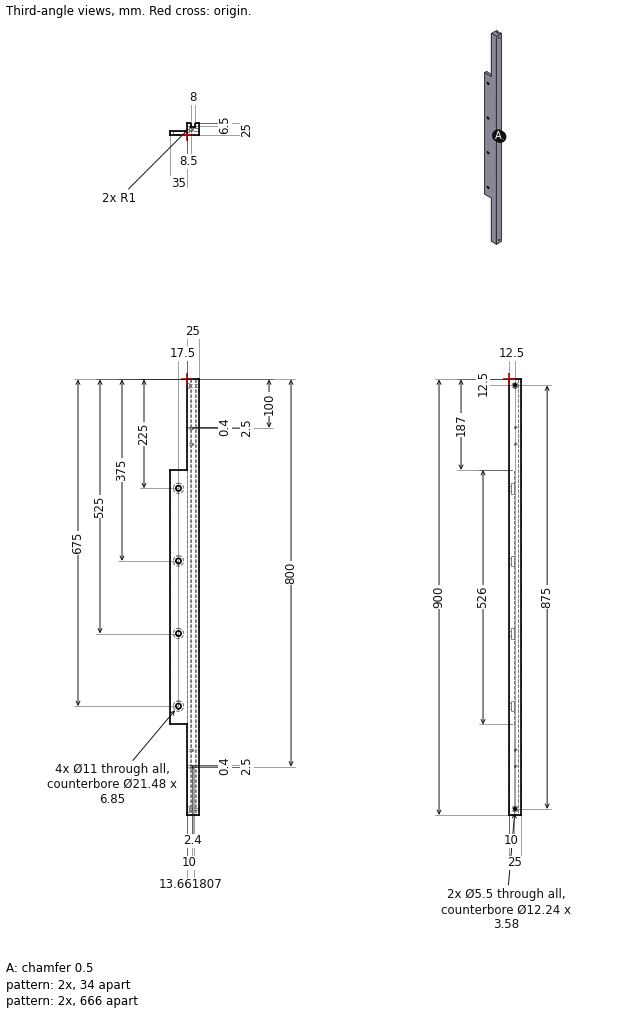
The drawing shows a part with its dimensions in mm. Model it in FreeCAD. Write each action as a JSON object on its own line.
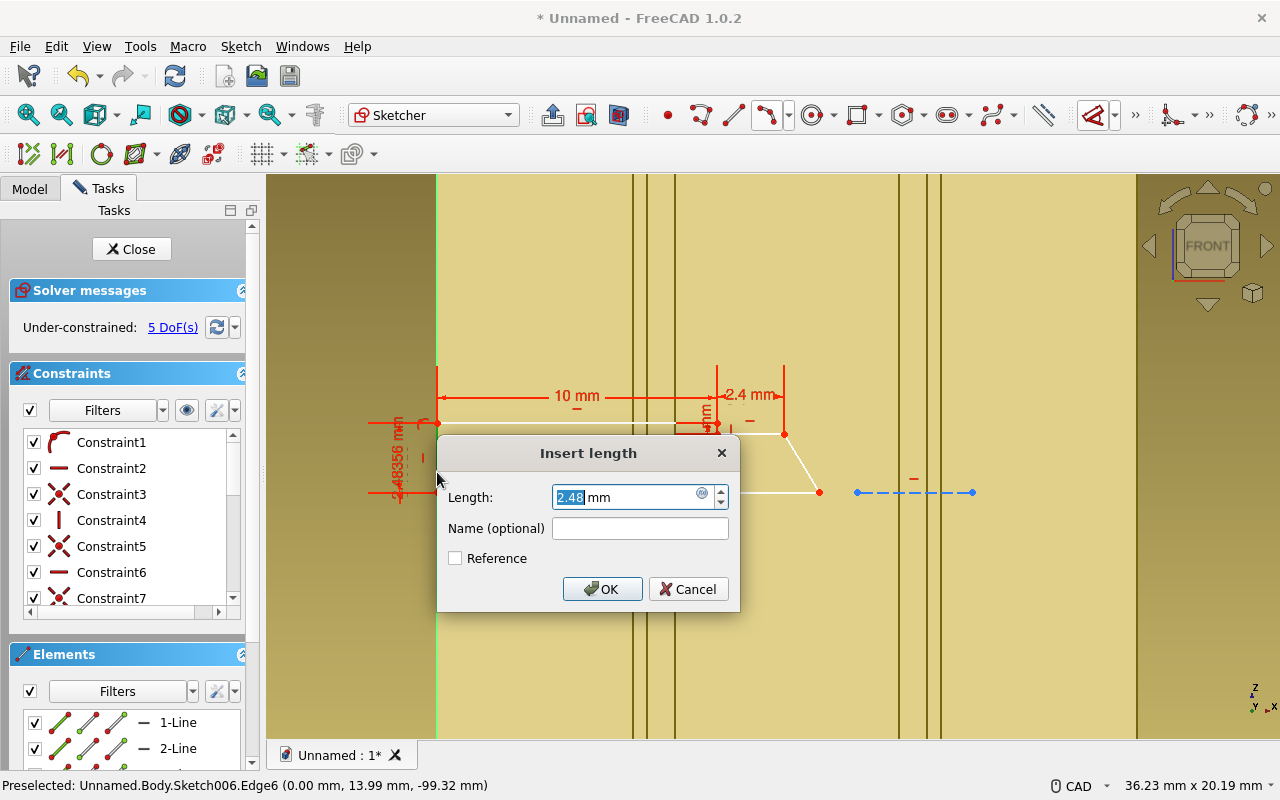
{"action": "type", "text": "2.5"}
{"action": "key", "text": "Return"}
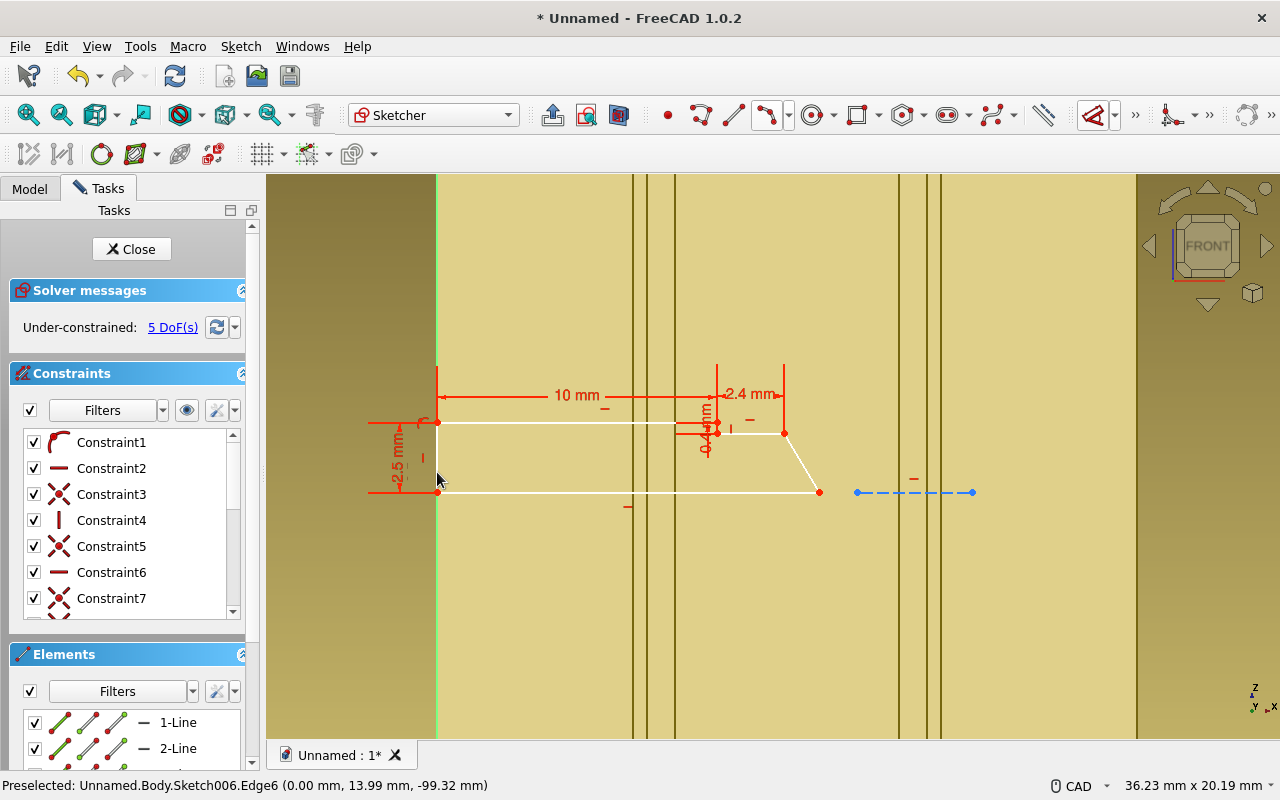
{"action": "left_click", "coordinate": [819, 493]}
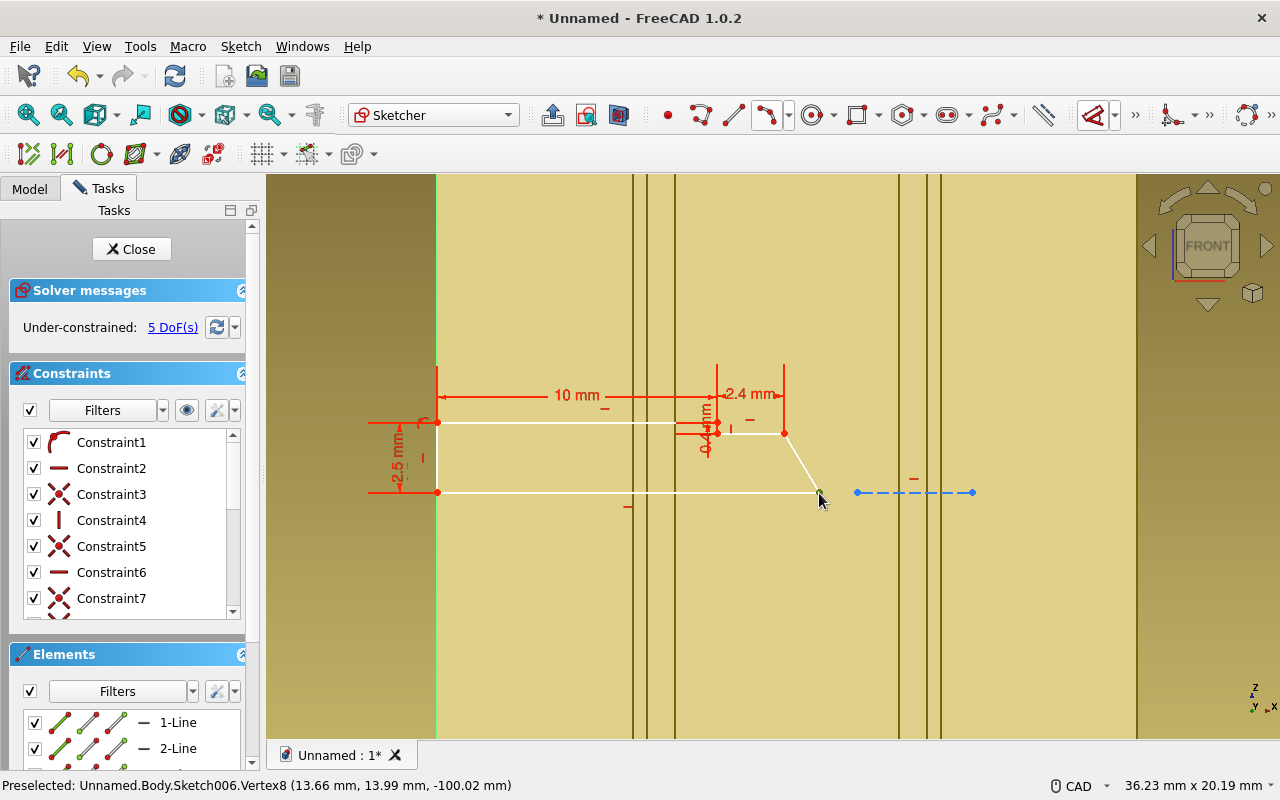
{"action": "left_click", "coordinate": [1114, 116]}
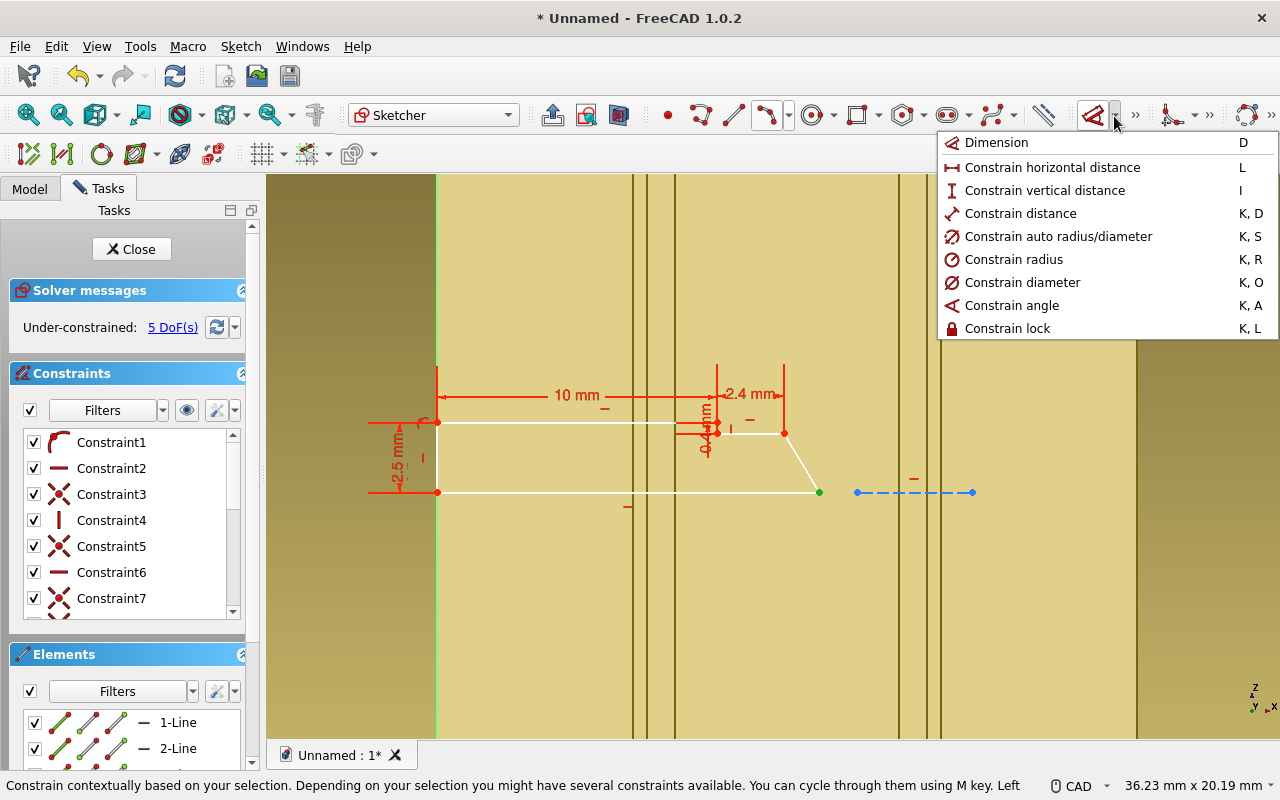
{"action": "left_click", "coordinate": [1108, 190]}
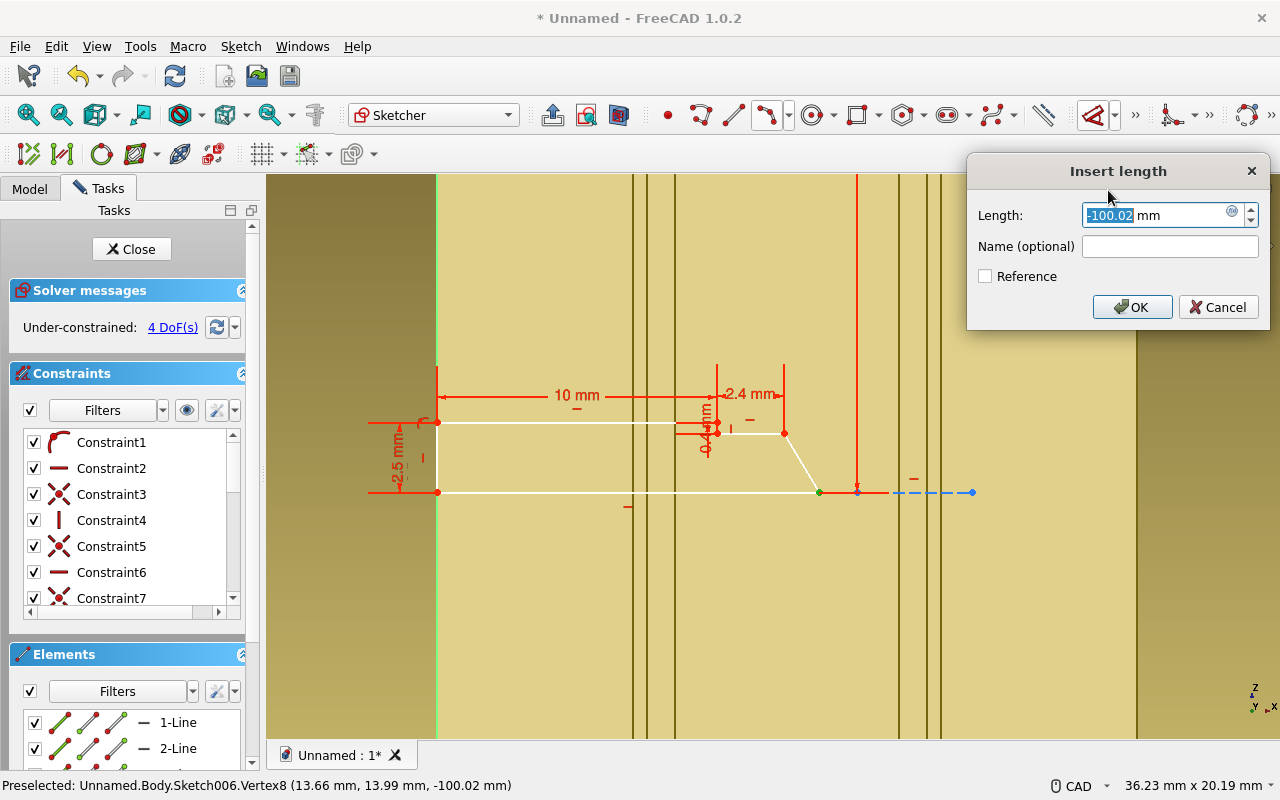
{"action": "type", "text": "-100"}
{"action": "key", "text": "Return"}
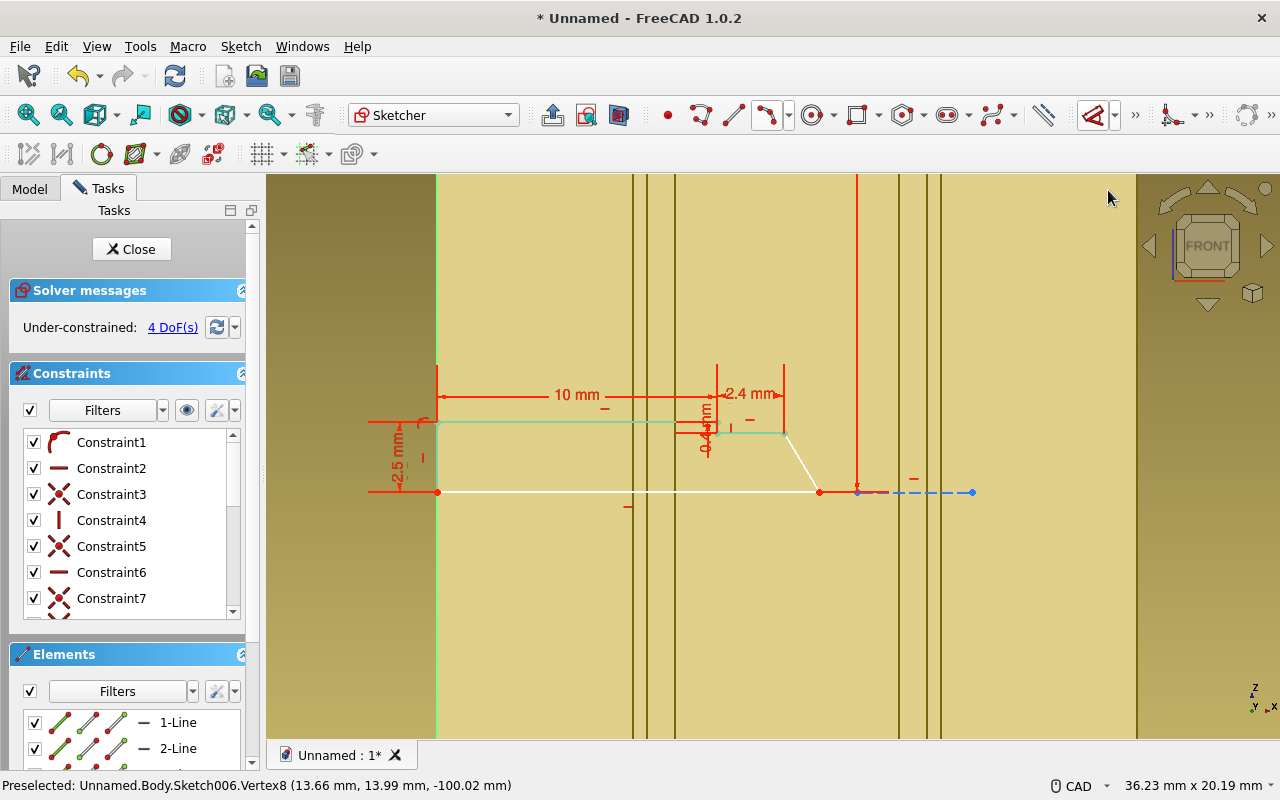
{"action": "left_click", "coordinate": [858, 493]}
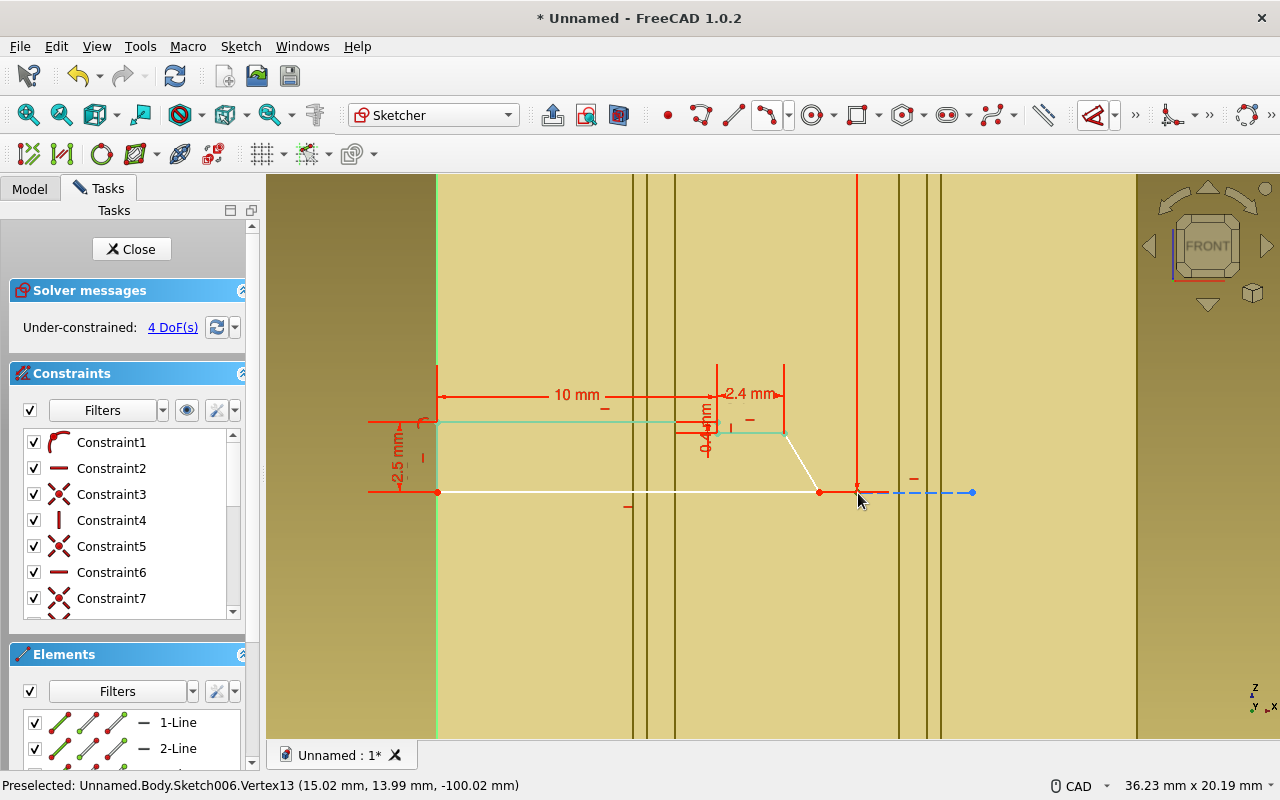
{"action": "key", "text": "i"}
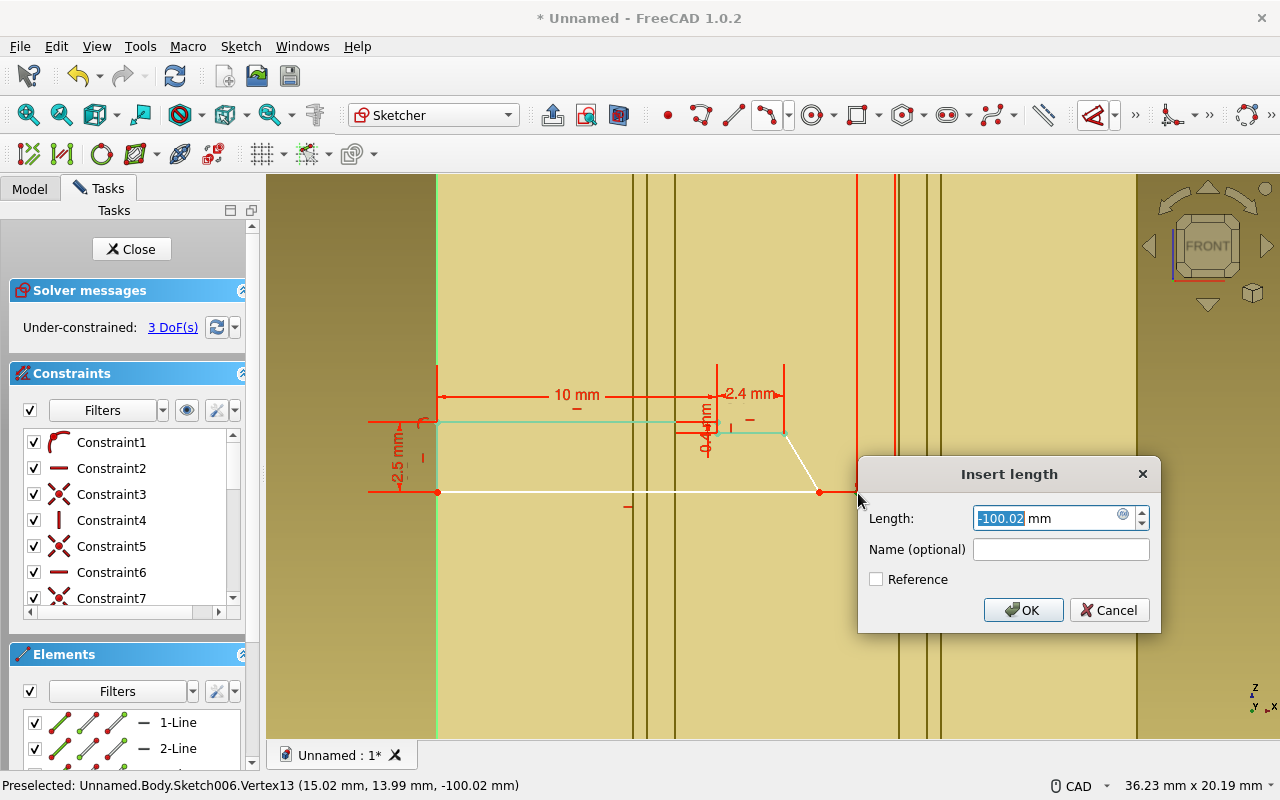
{"action": "type", "text": "-100"}
{"action": "key", "text": "Return"}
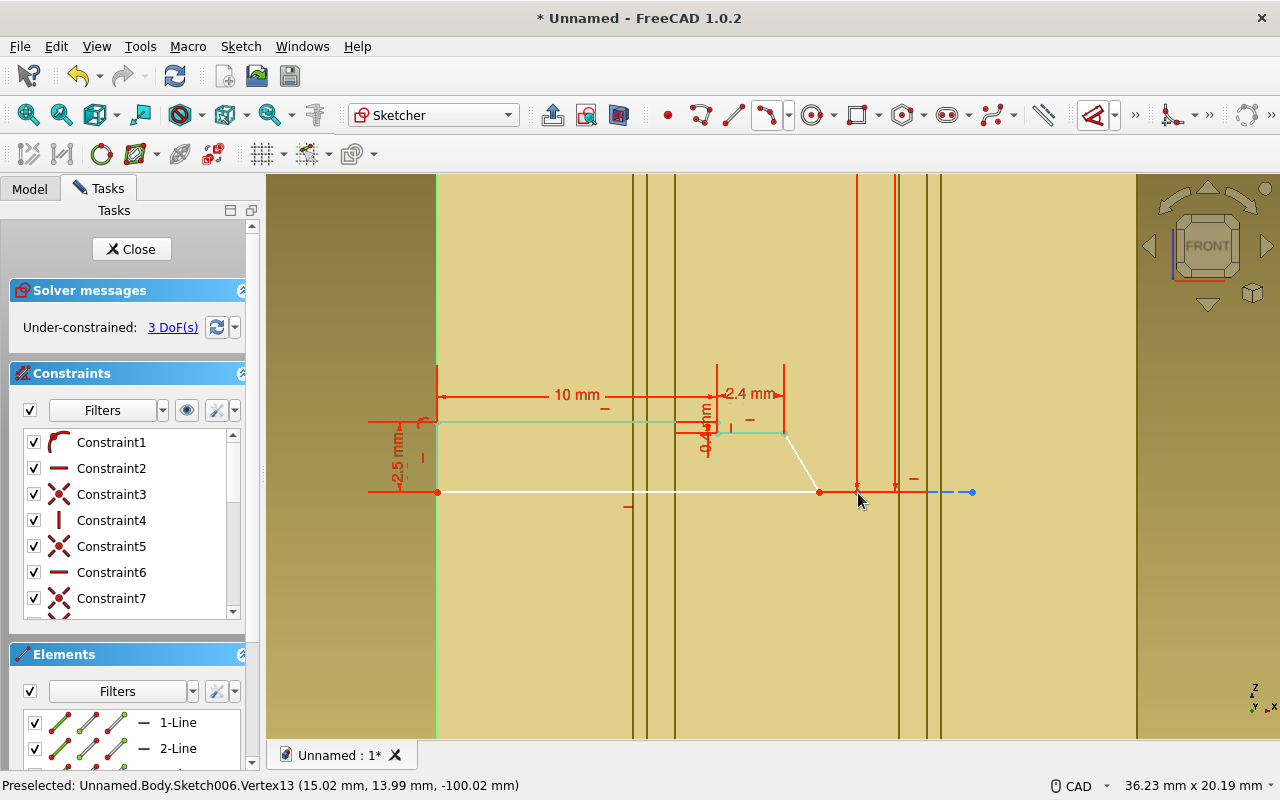
{"action": "left_click", "coordinate": [705, 492]}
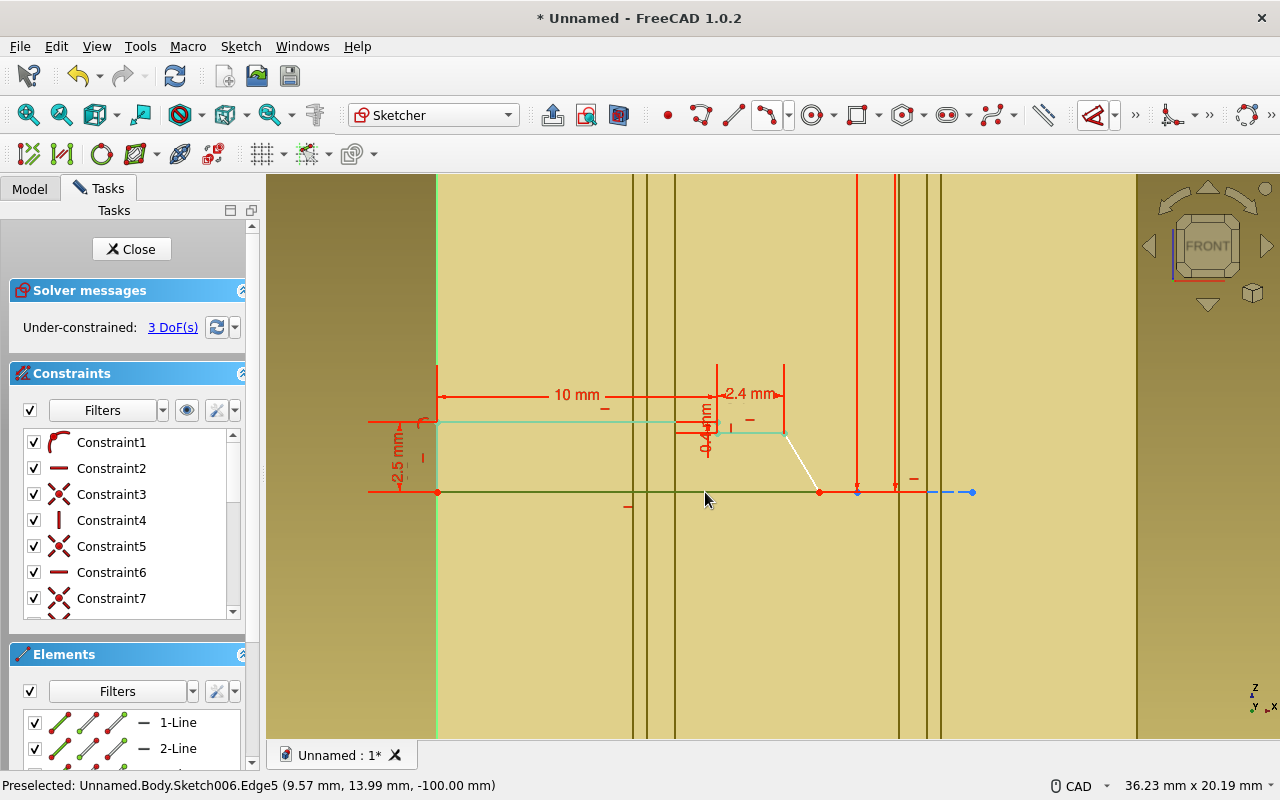
{"action": "left_click", "coordinate": [1114, 116]}